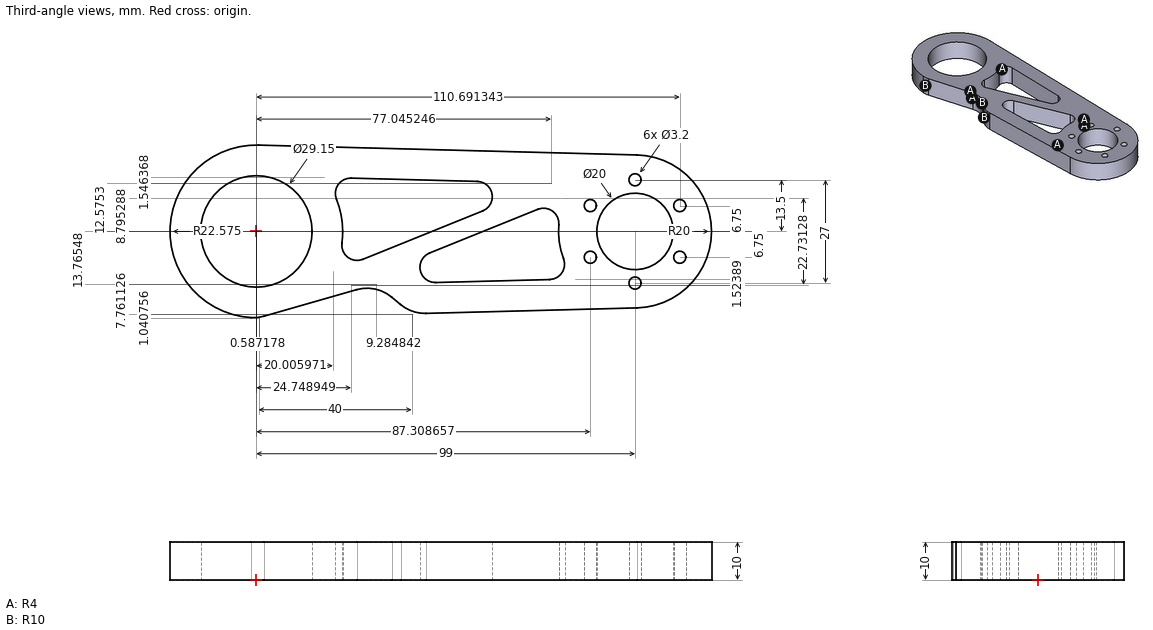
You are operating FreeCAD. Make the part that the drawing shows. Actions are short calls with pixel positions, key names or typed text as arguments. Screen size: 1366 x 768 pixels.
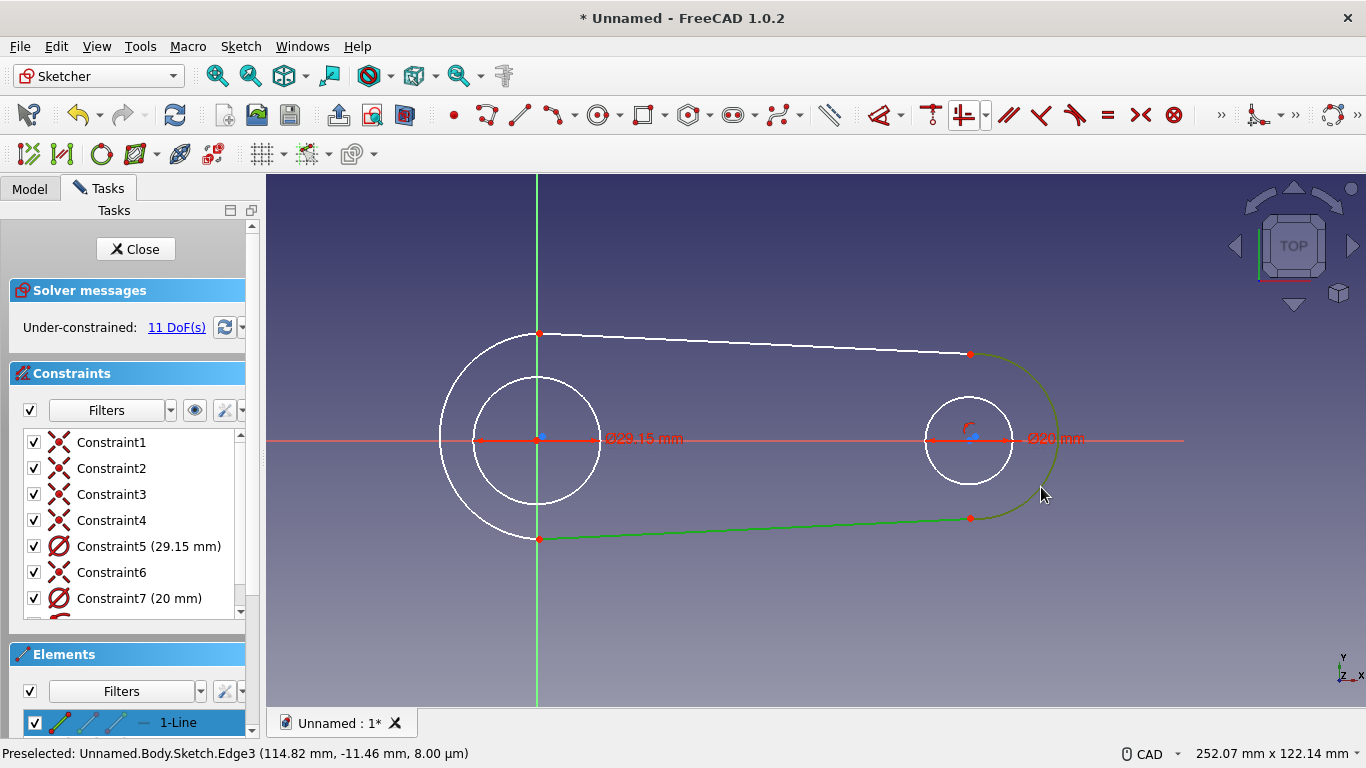
key(t)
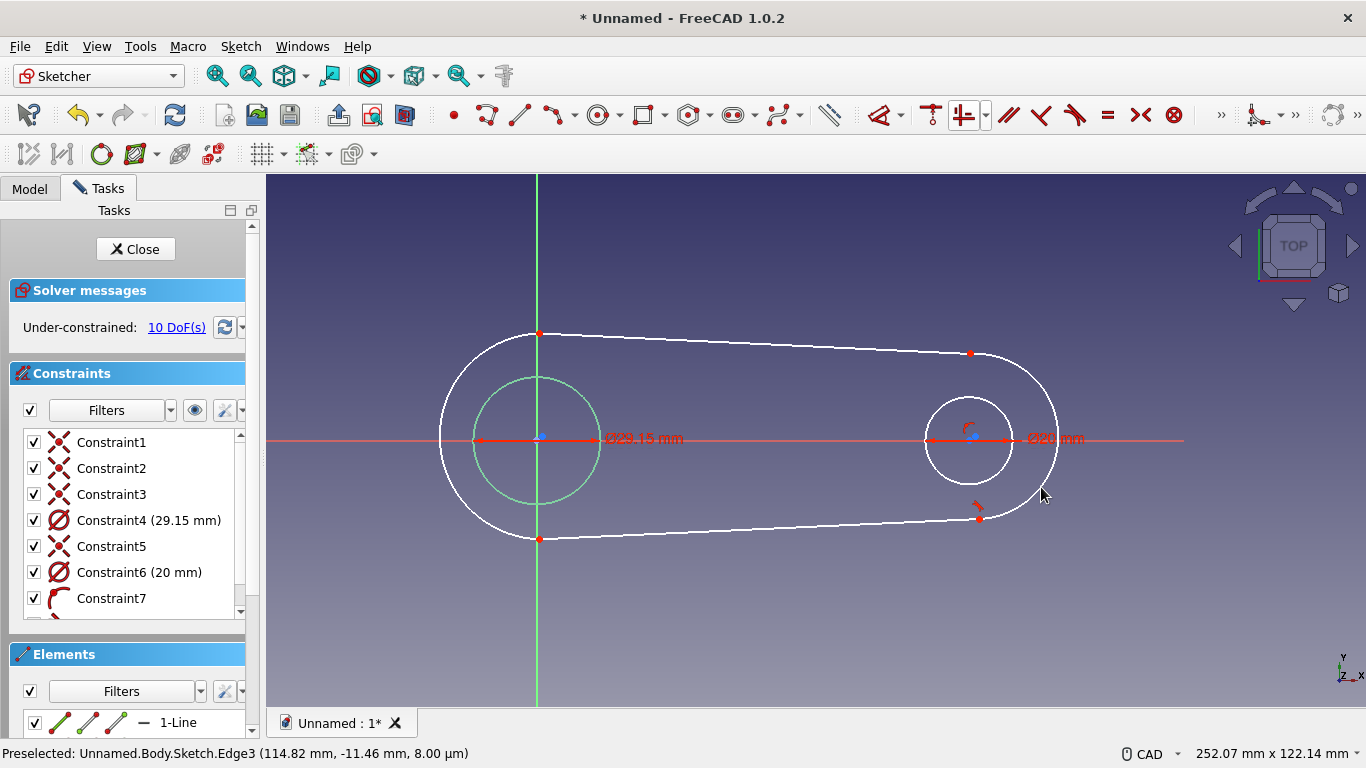
click(671, 533)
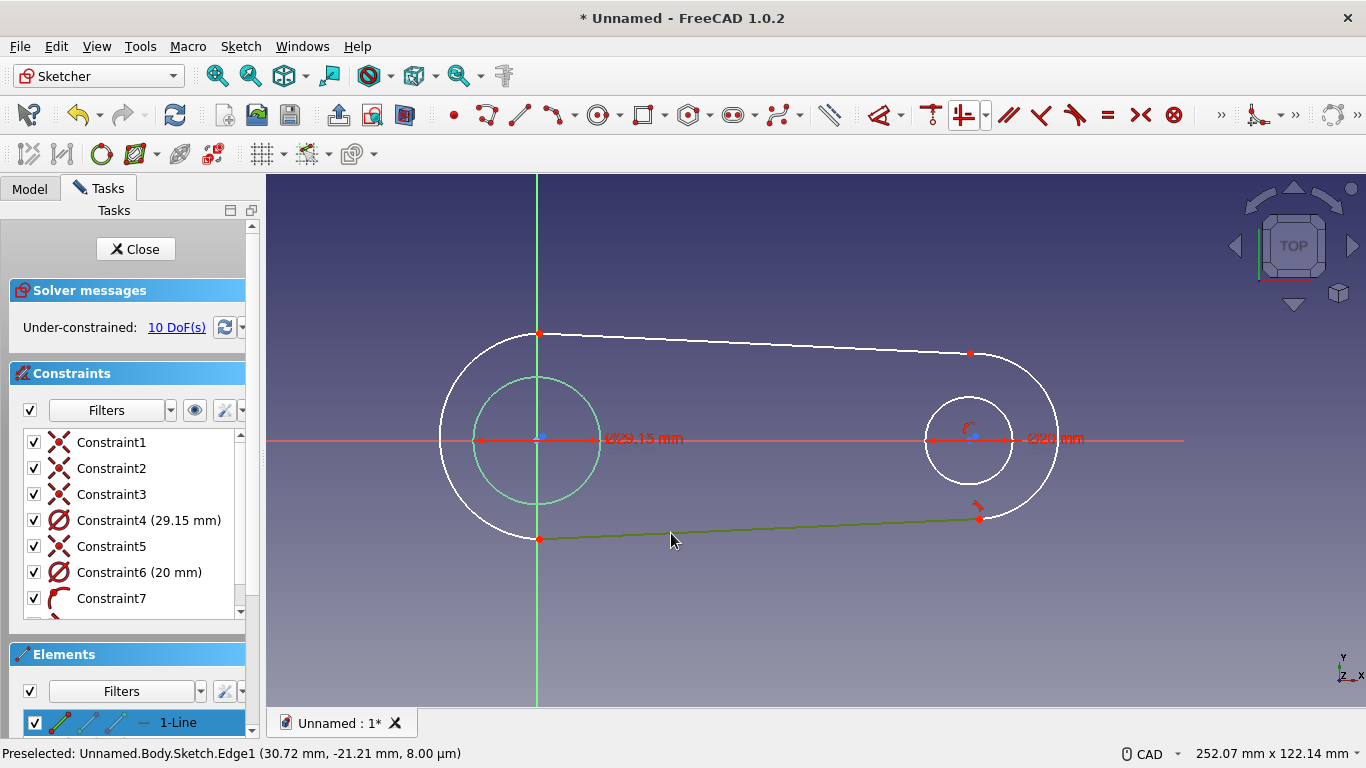
click(459, 377)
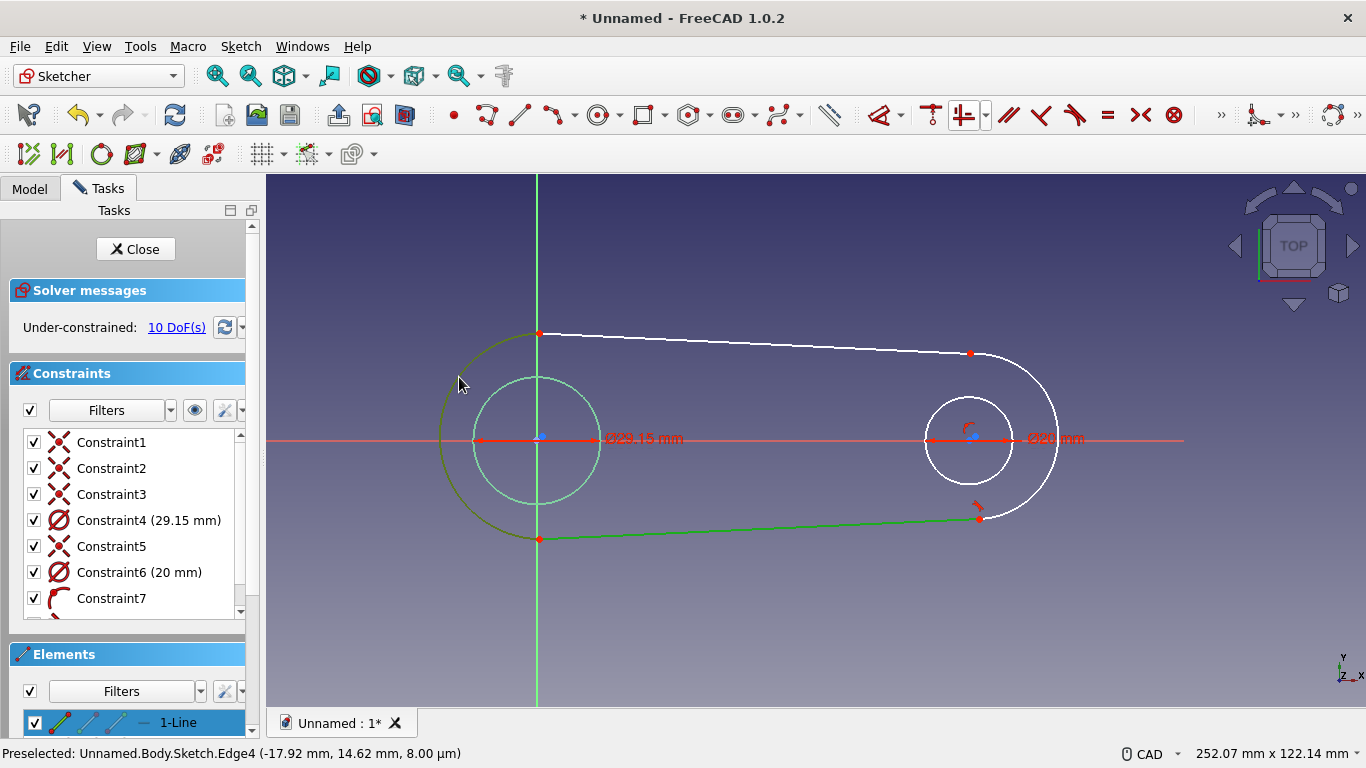
key(t)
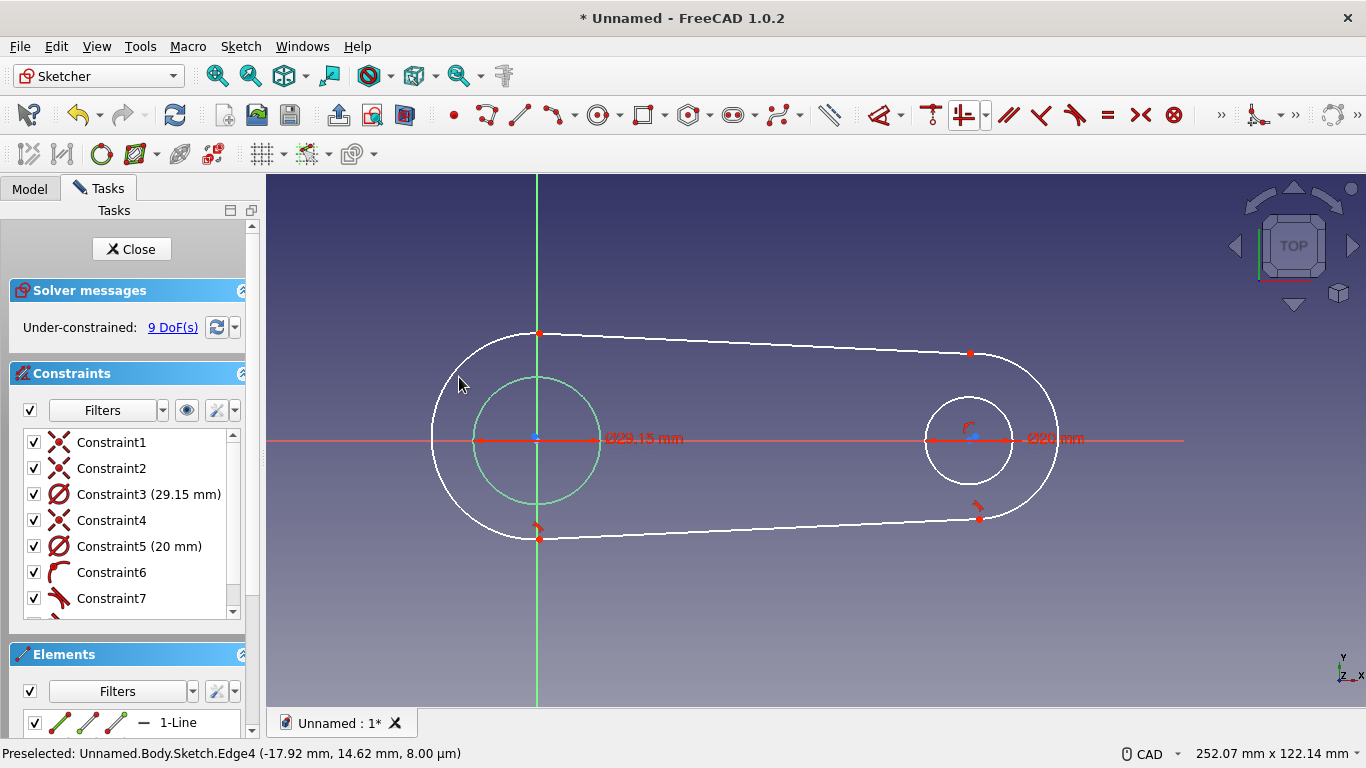
click(842, 348)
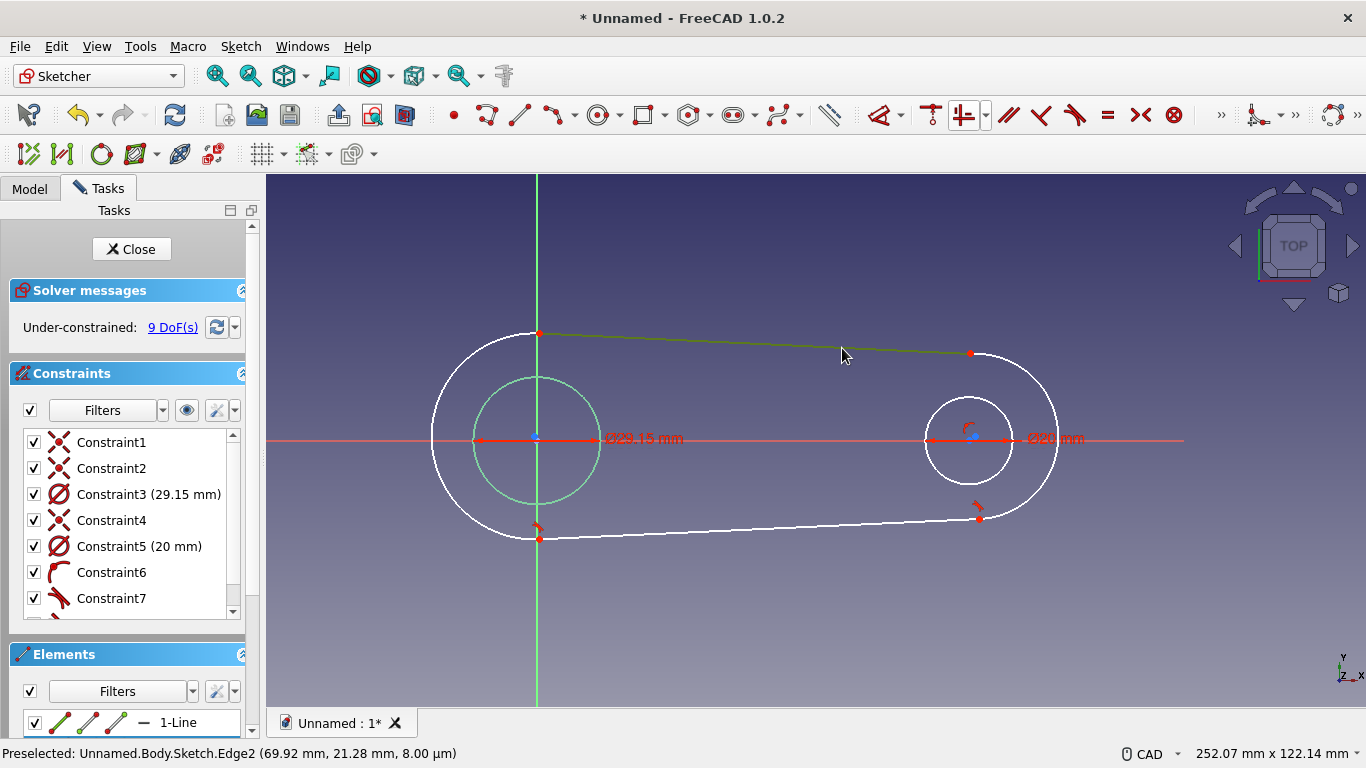
click(1045, 482)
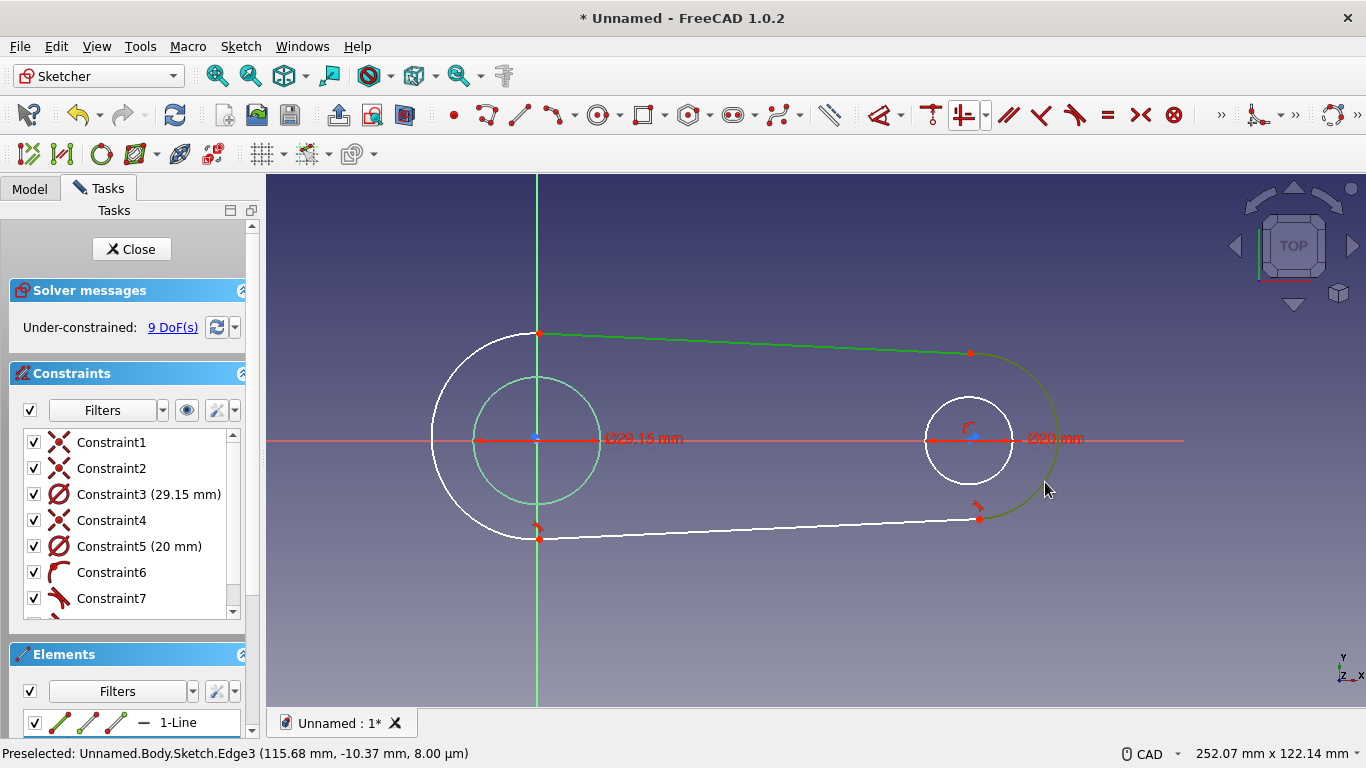
click(1075, 116)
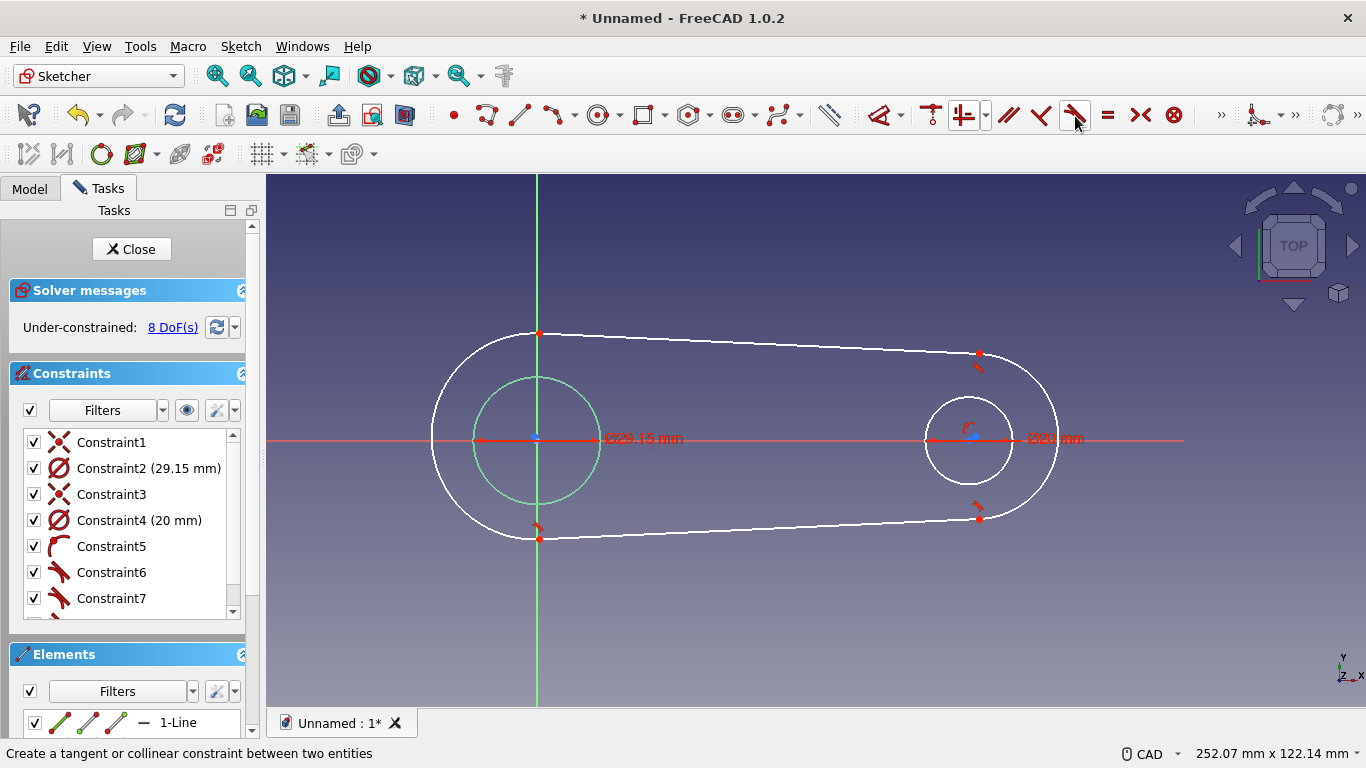
click(847, 348)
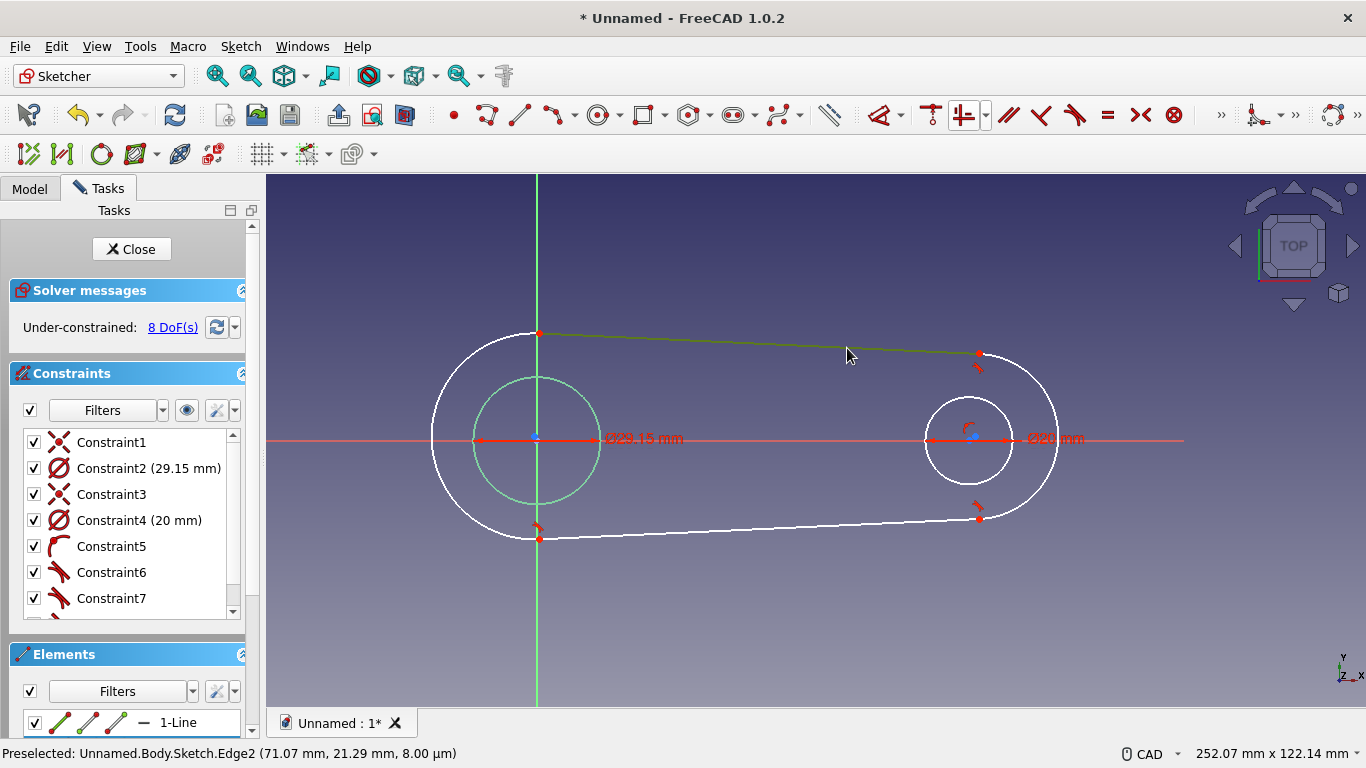
click(452, 374)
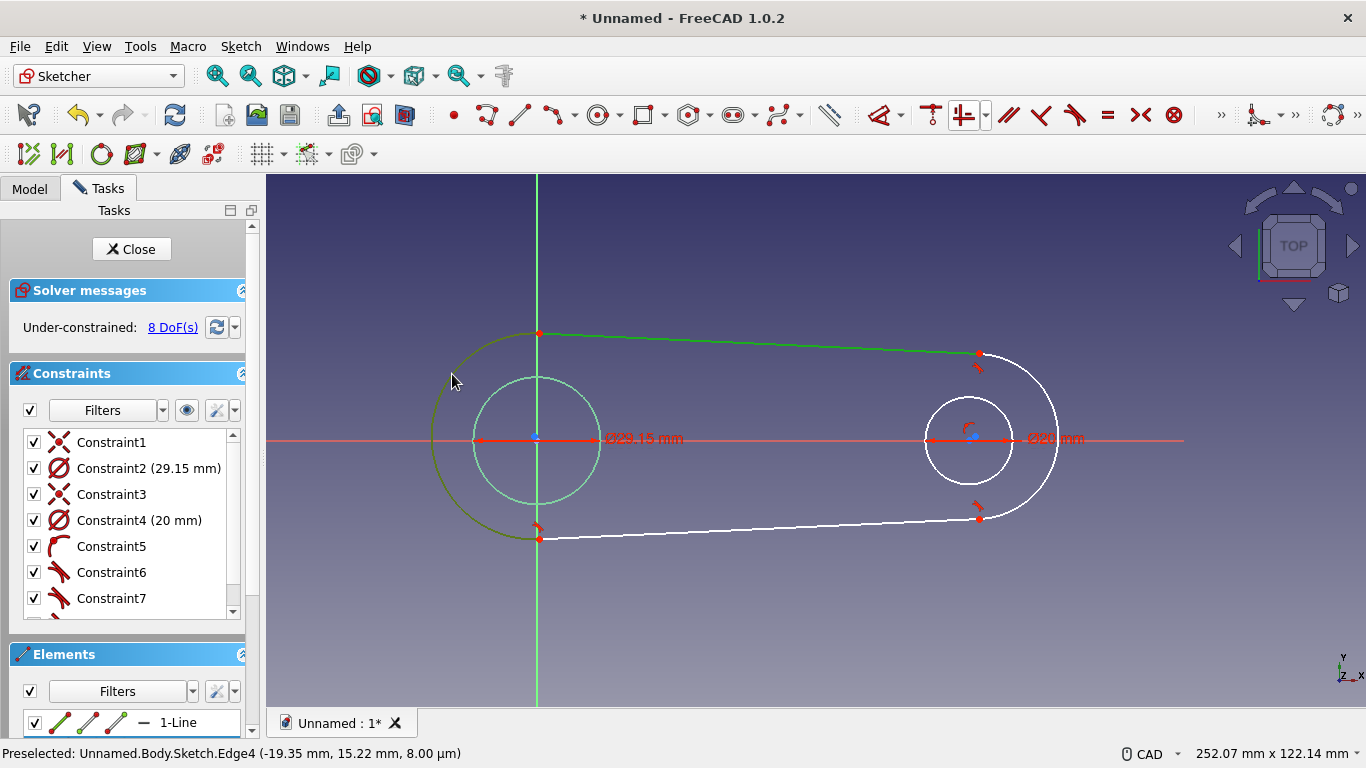
click(1075, 116)